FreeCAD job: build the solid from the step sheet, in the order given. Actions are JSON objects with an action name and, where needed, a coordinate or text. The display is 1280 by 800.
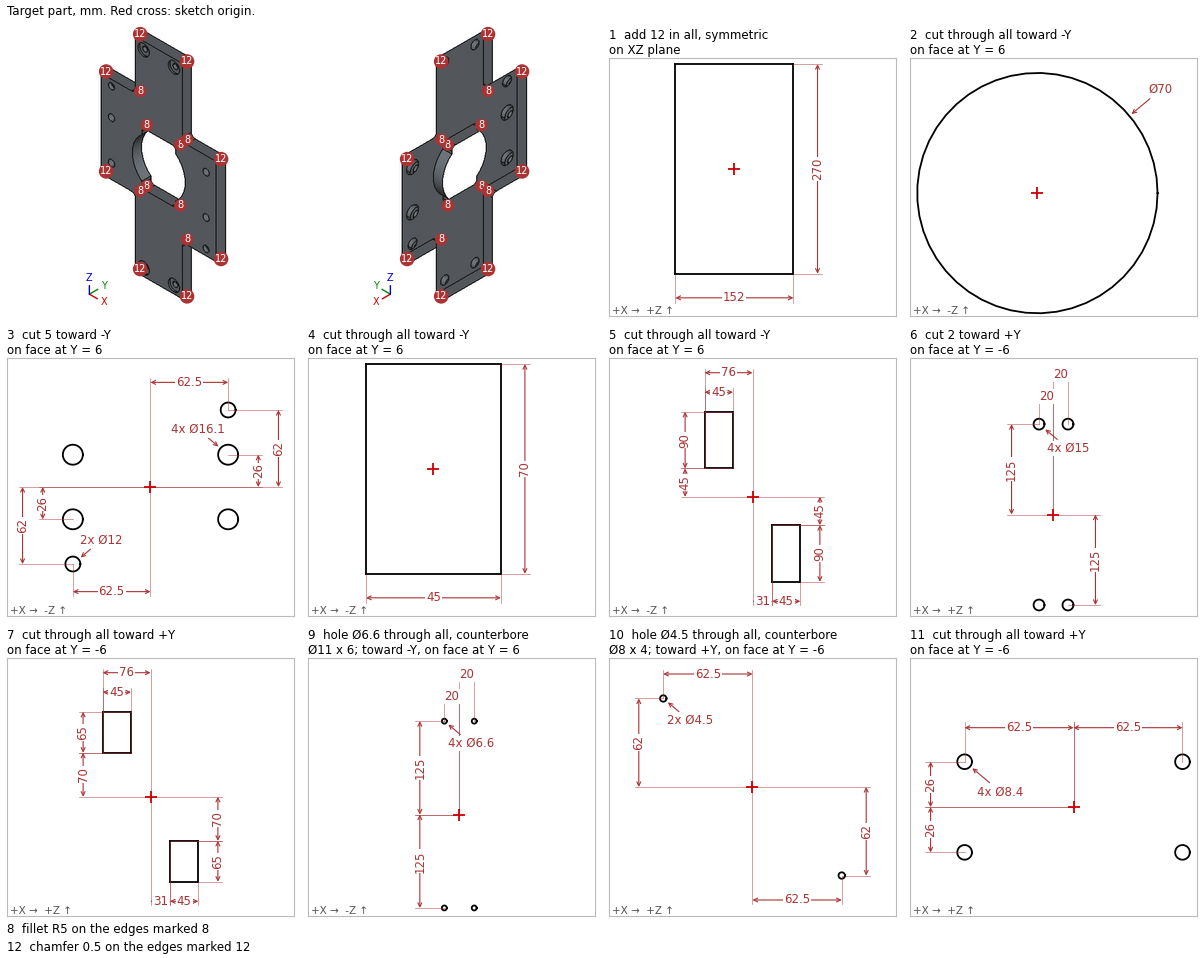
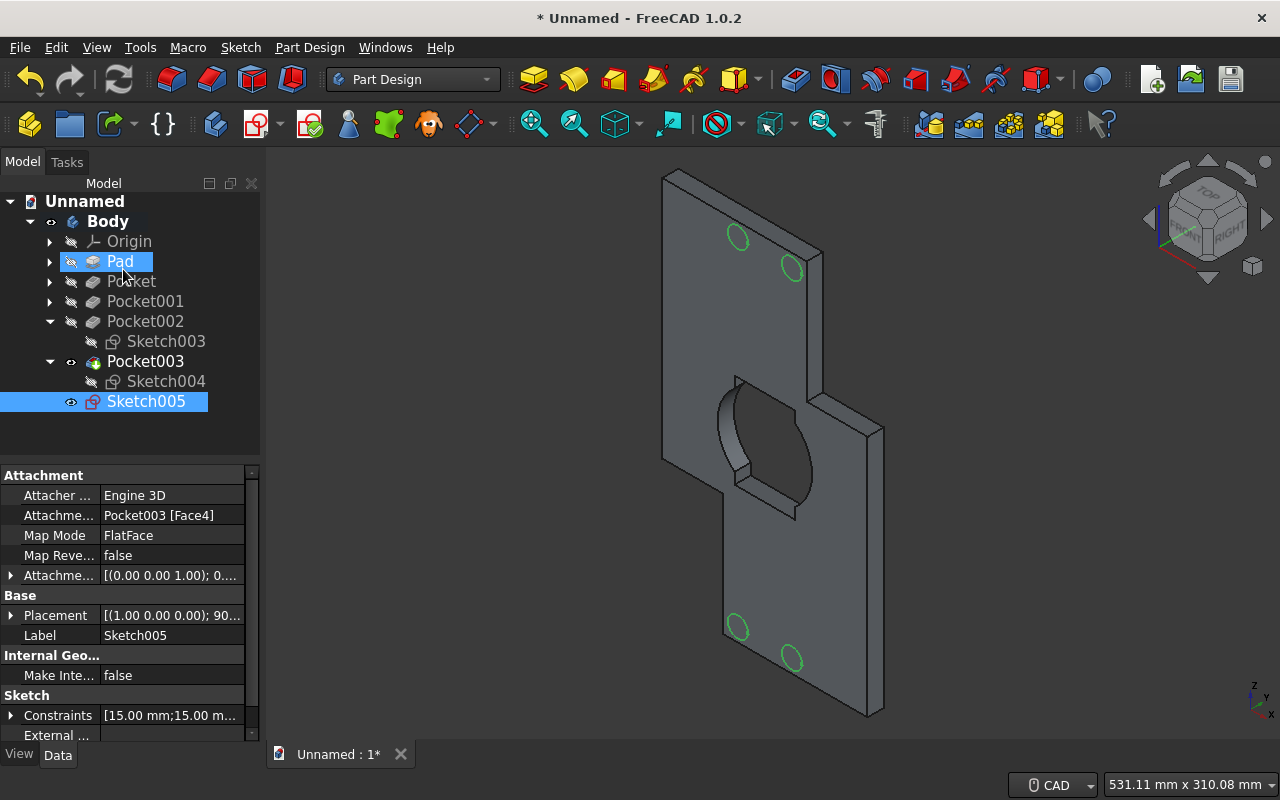
{"action": "left_click", "coordinate": [796, 80]}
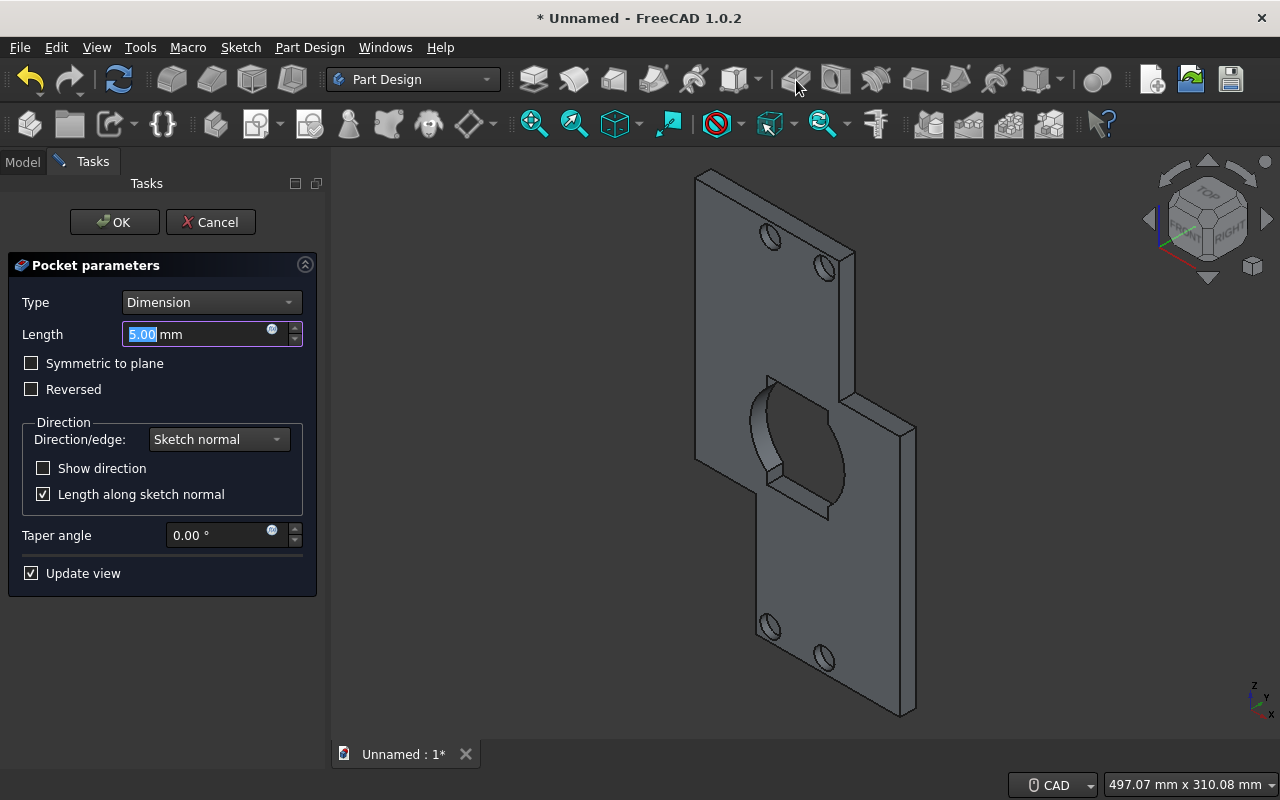
{"action": "type", "text": "2"}
{"action": "key", "text": "Tab"}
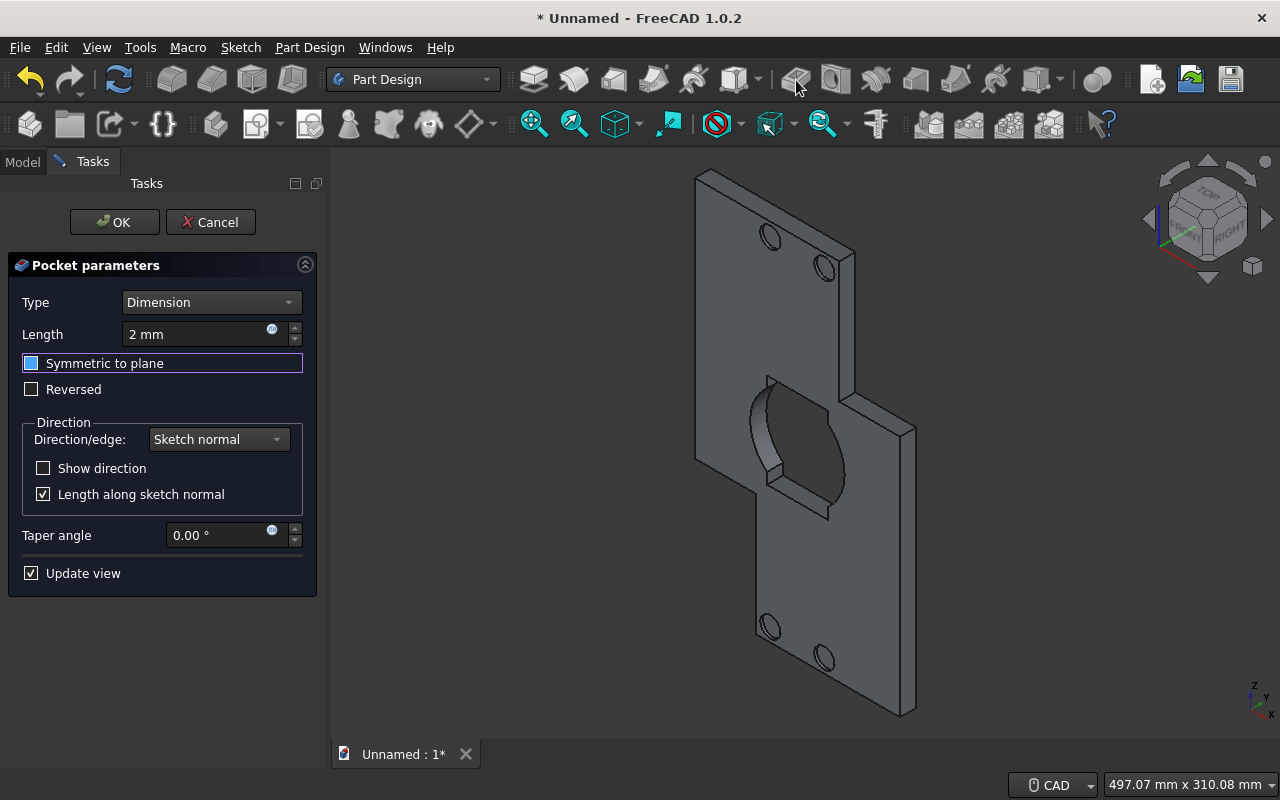
{"action": "left_click", "coordinate": [115, 222]}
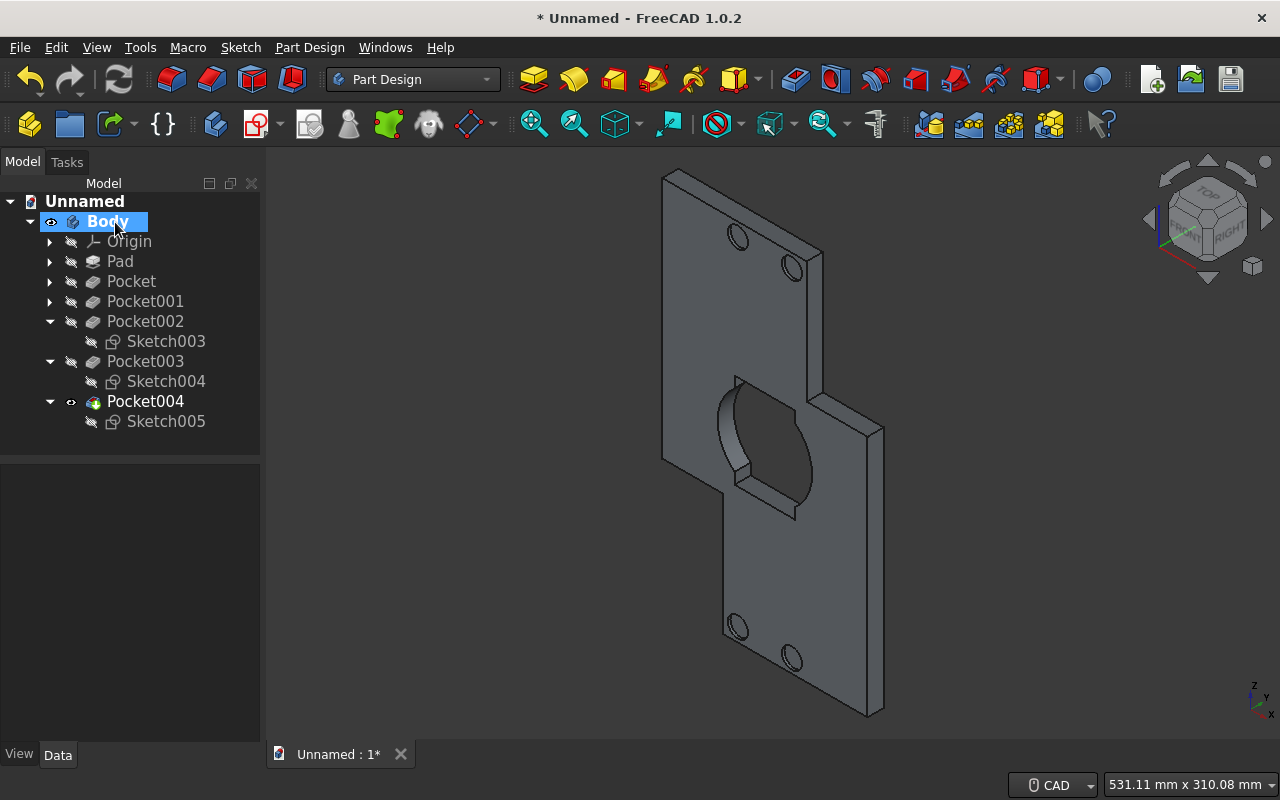
{"action": "left_click", "coordinate": [794, 584]}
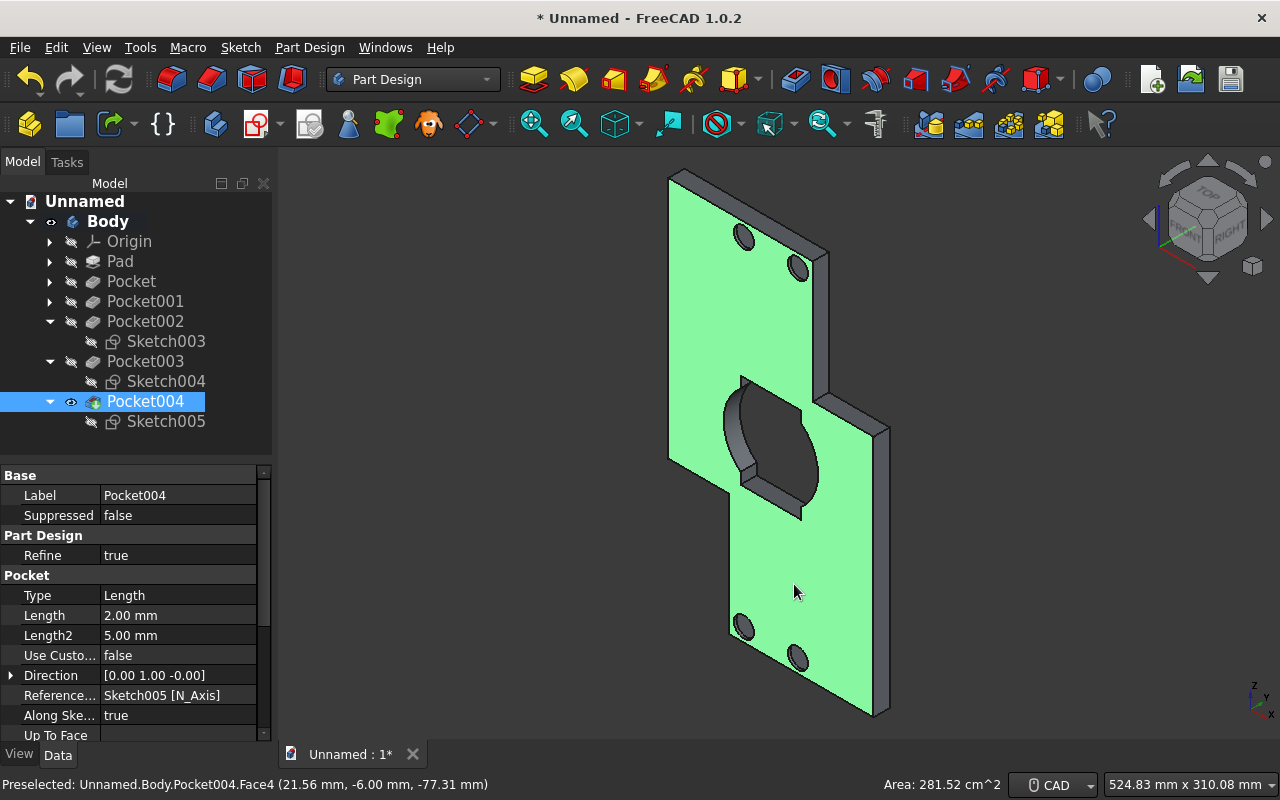
{"action": "left_click", "coordinate": [256, 124]}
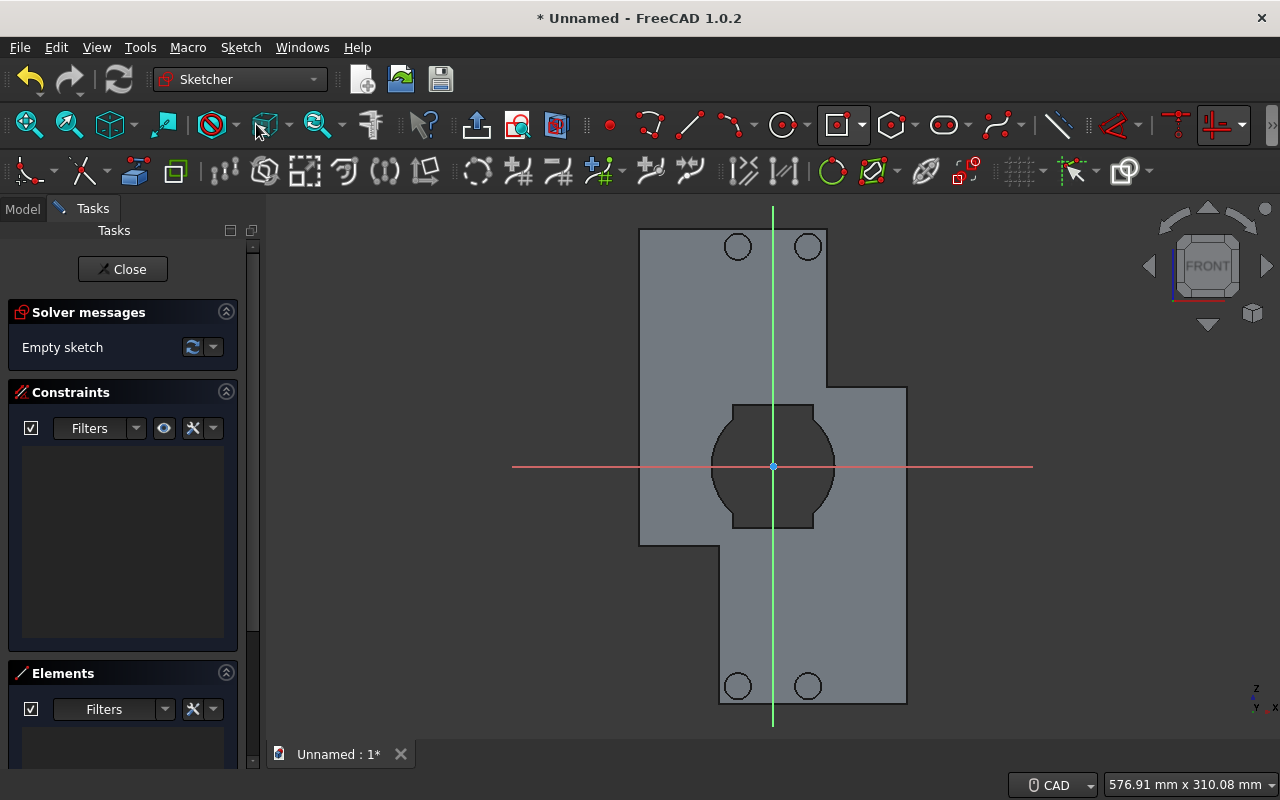
{"action": "scroll", "coordinate": [565, 466], "scroll_direction": "down", "scroll_amount": 2}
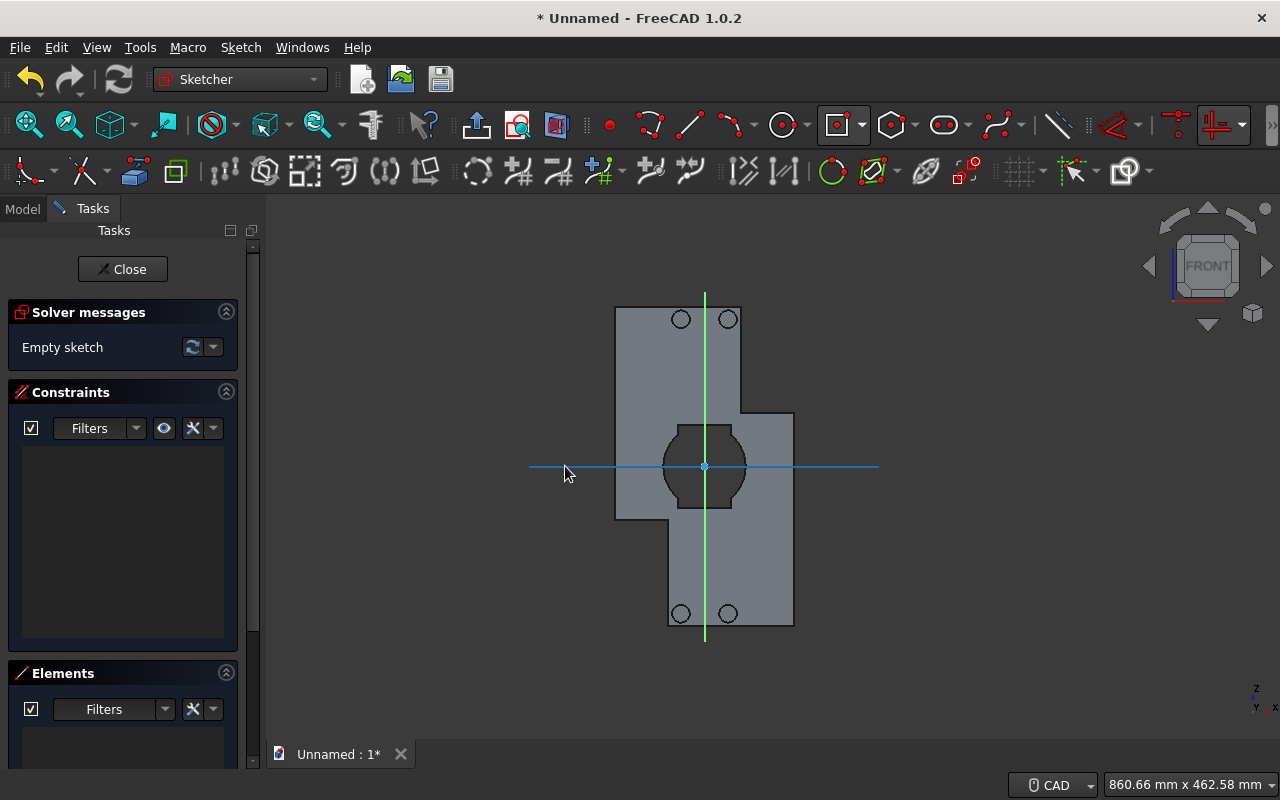
{"action": "key", "text": "g r"}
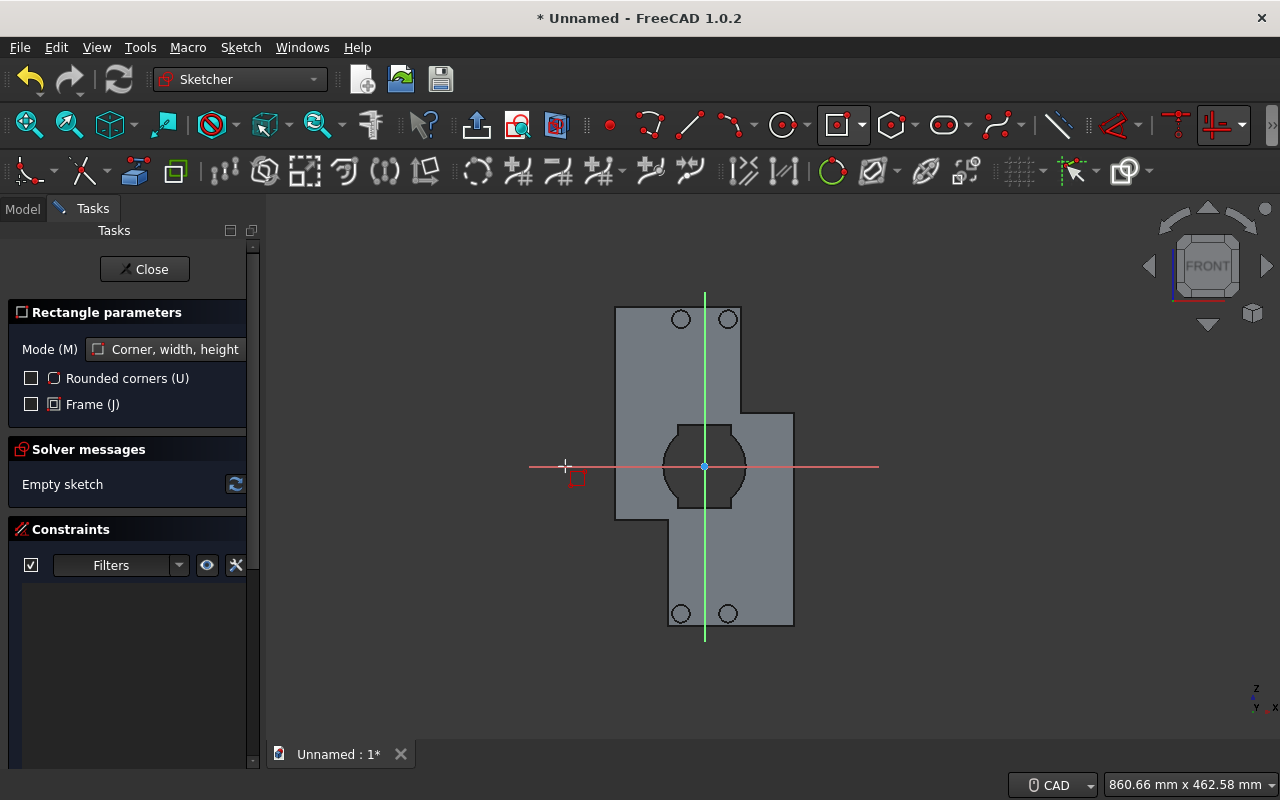
{"action": "left_click", "coordinate": [615, 307]}
{"action": "mouse_move", "coordinate": [668, 384]}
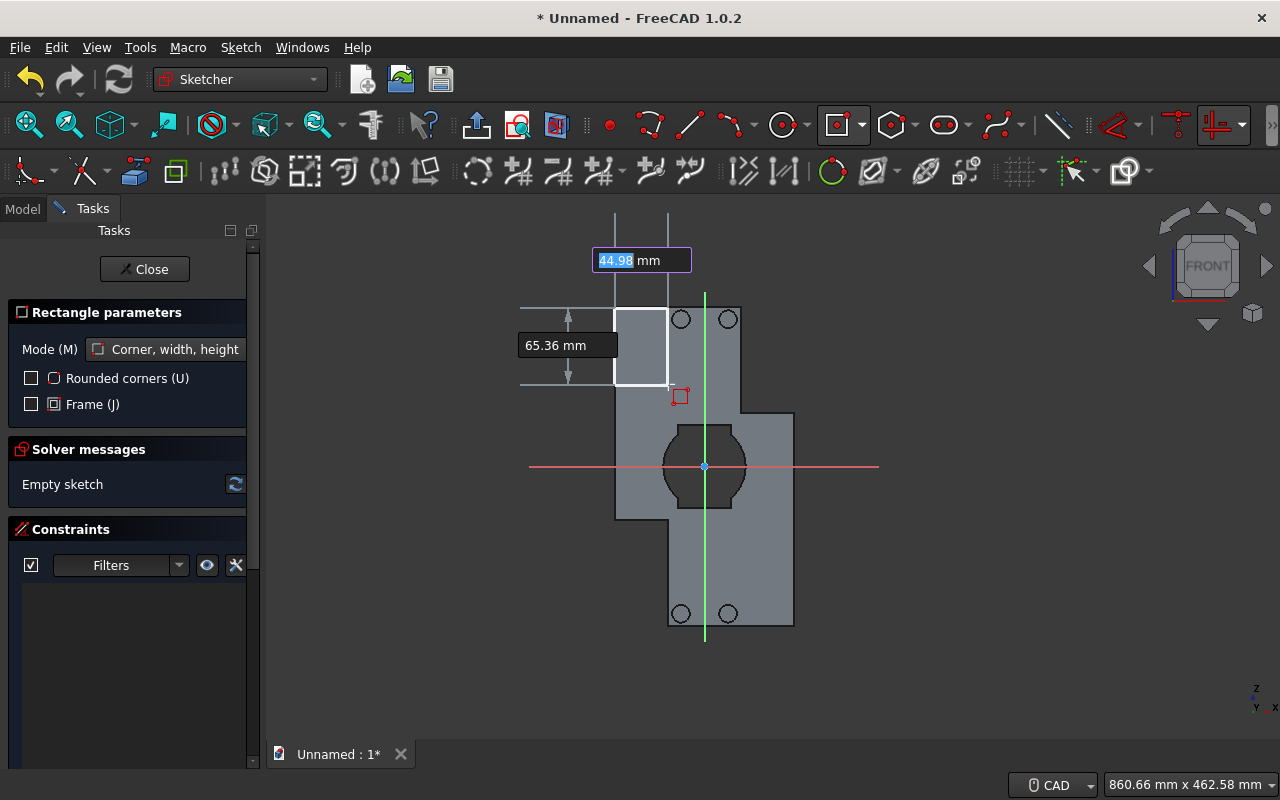
{"action": "type", "text": "45"}
{"action": "key", "text": "Tab"}
{"action": "type", "text": "65"}
{"action": "key", "text": "Return"}